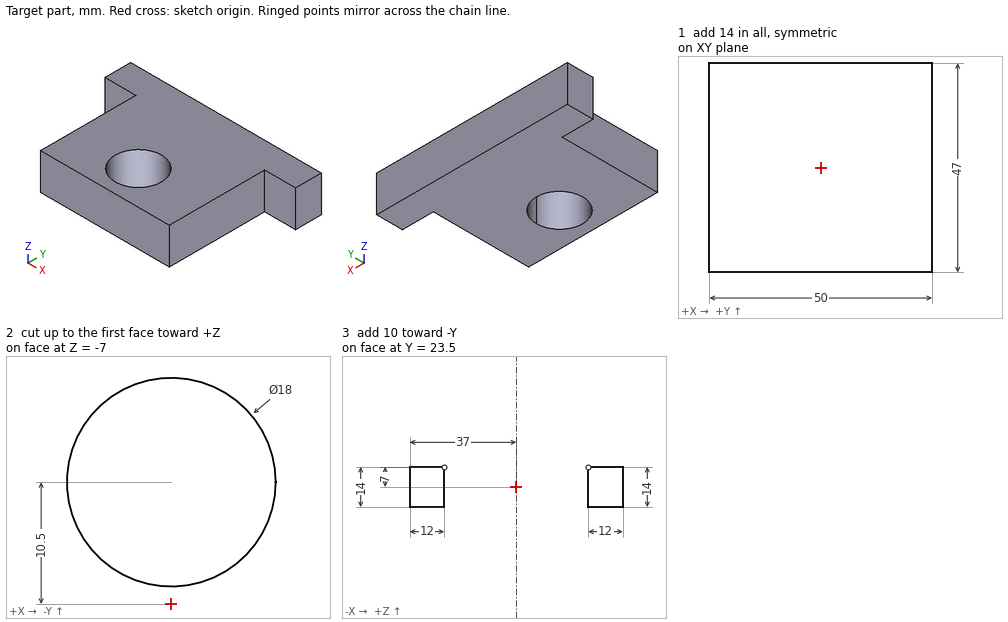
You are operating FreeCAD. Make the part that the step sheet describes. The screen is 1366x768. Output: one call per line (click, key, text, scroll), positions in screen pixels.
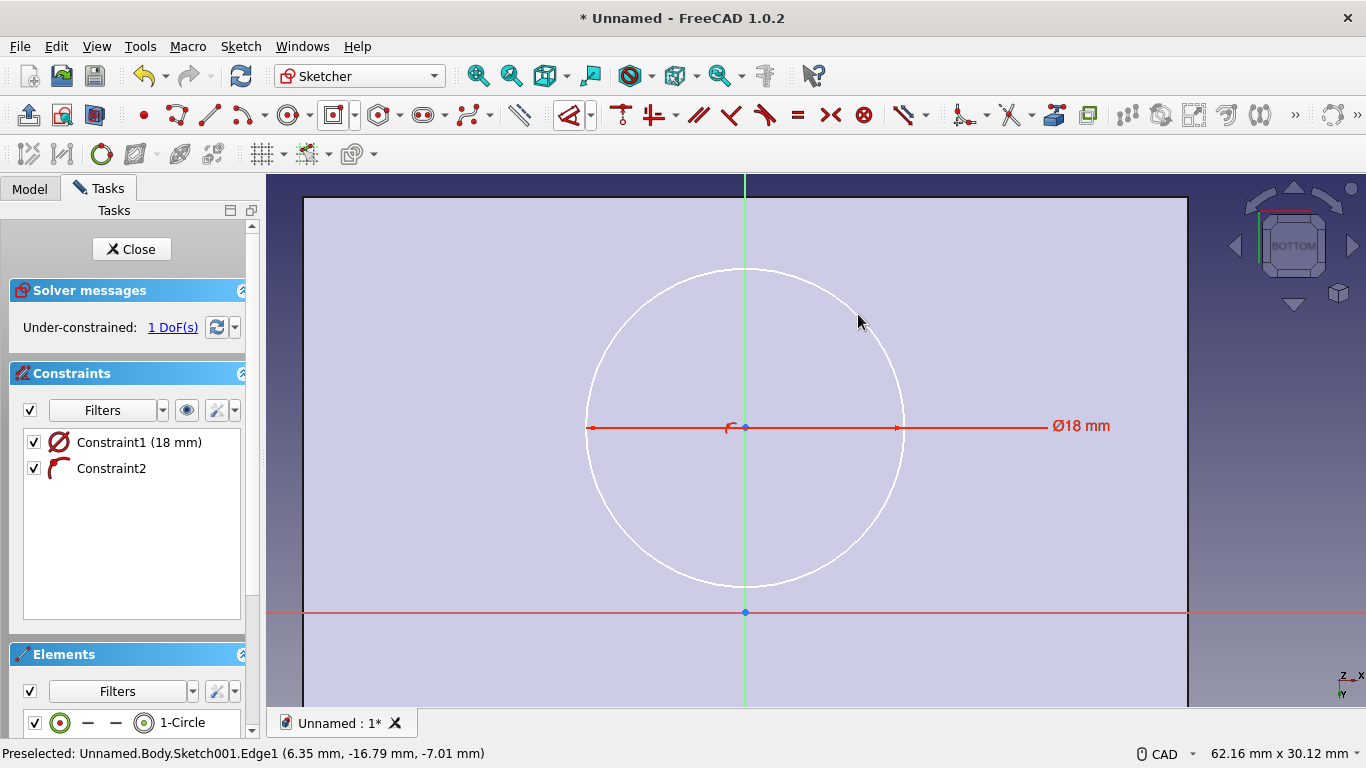
click(745, 428)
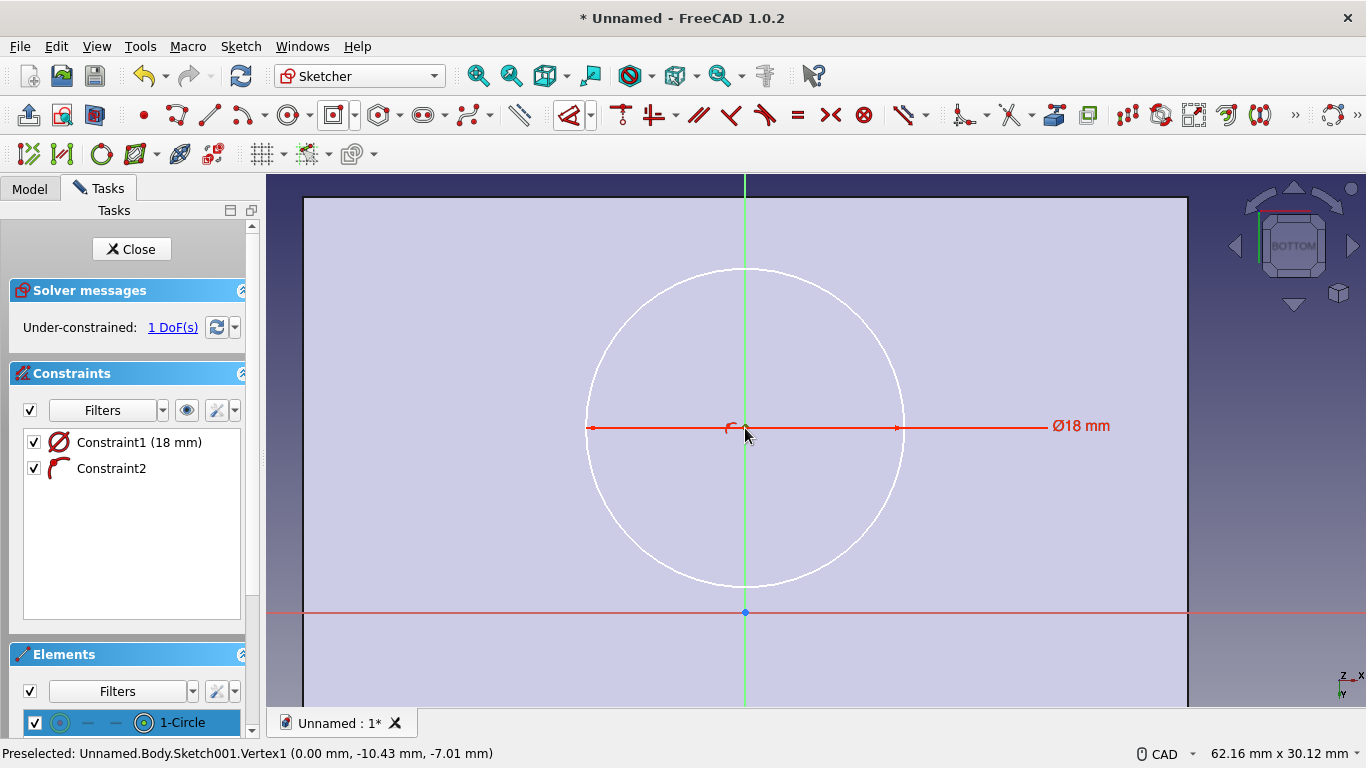
click(590, 116)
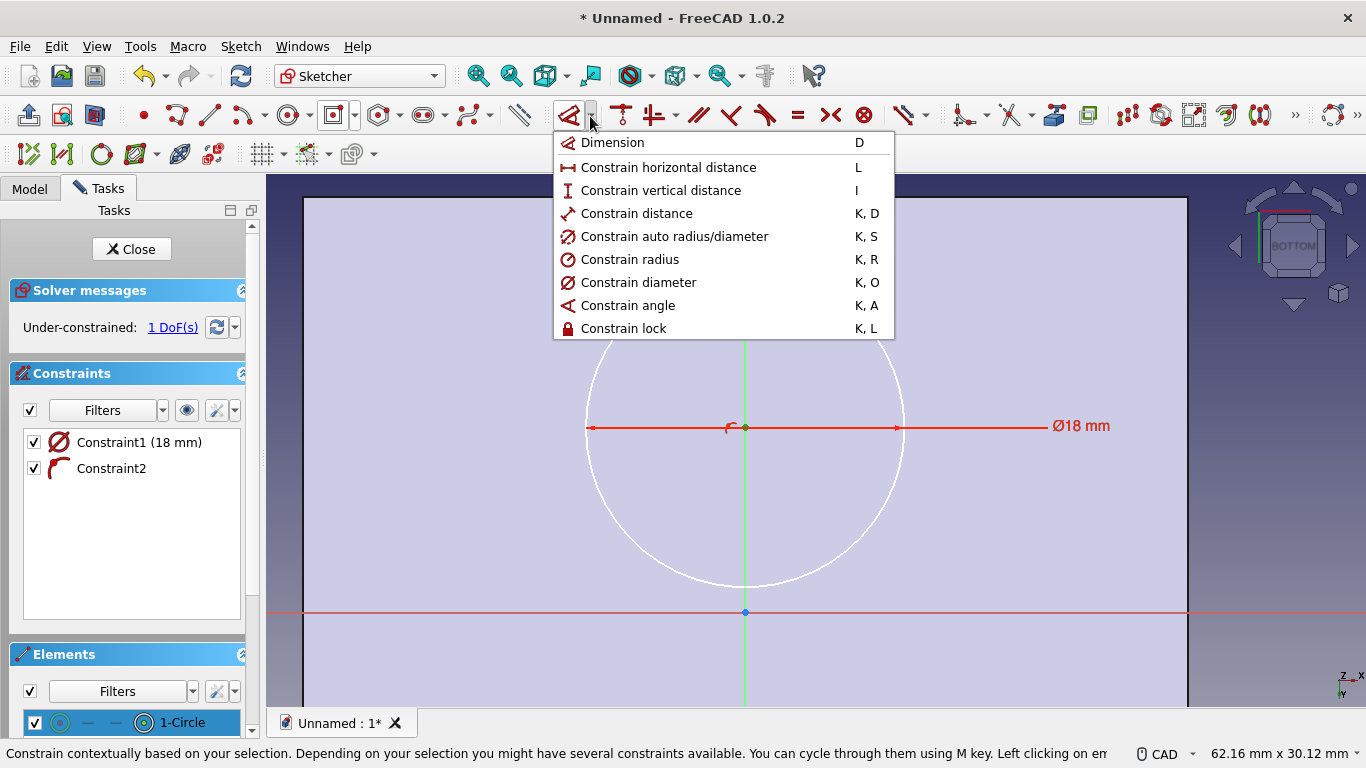
click(724, 190)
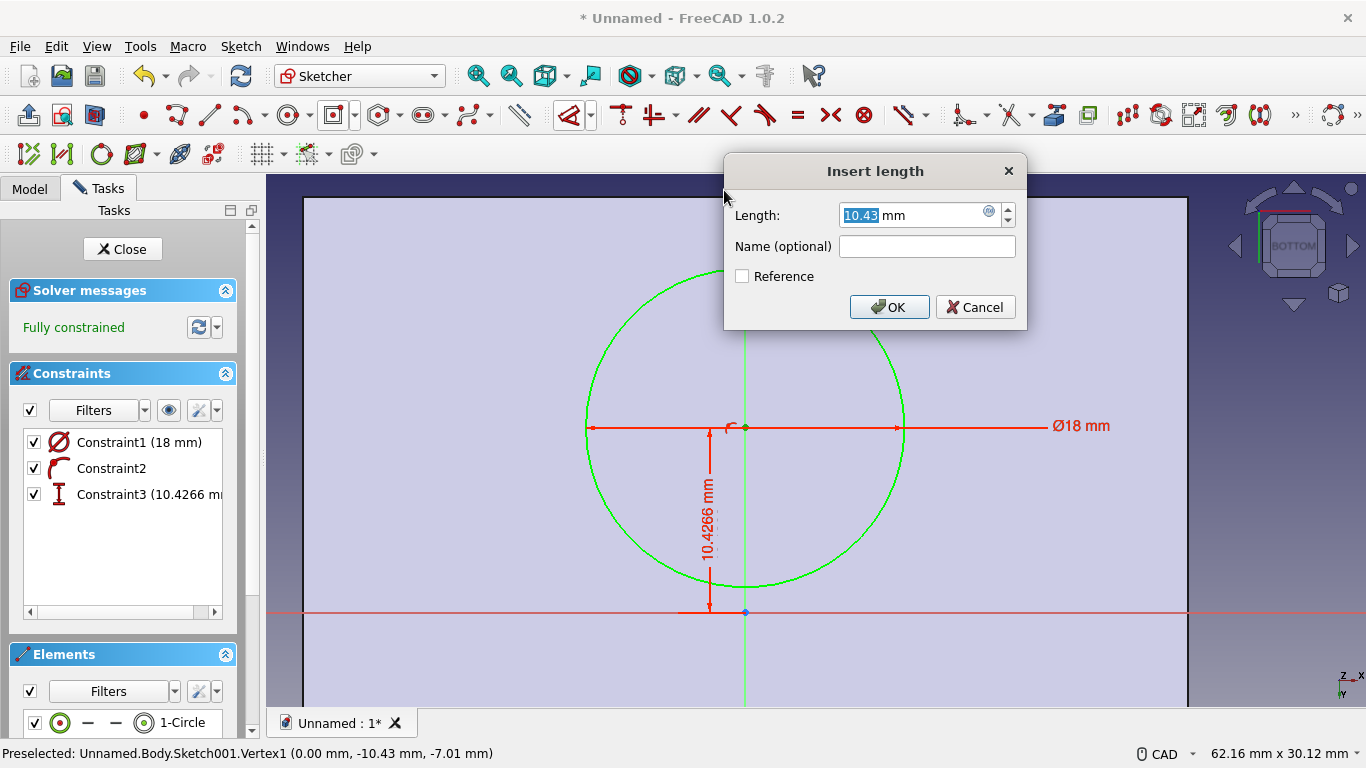
text(10.5)
key(Return)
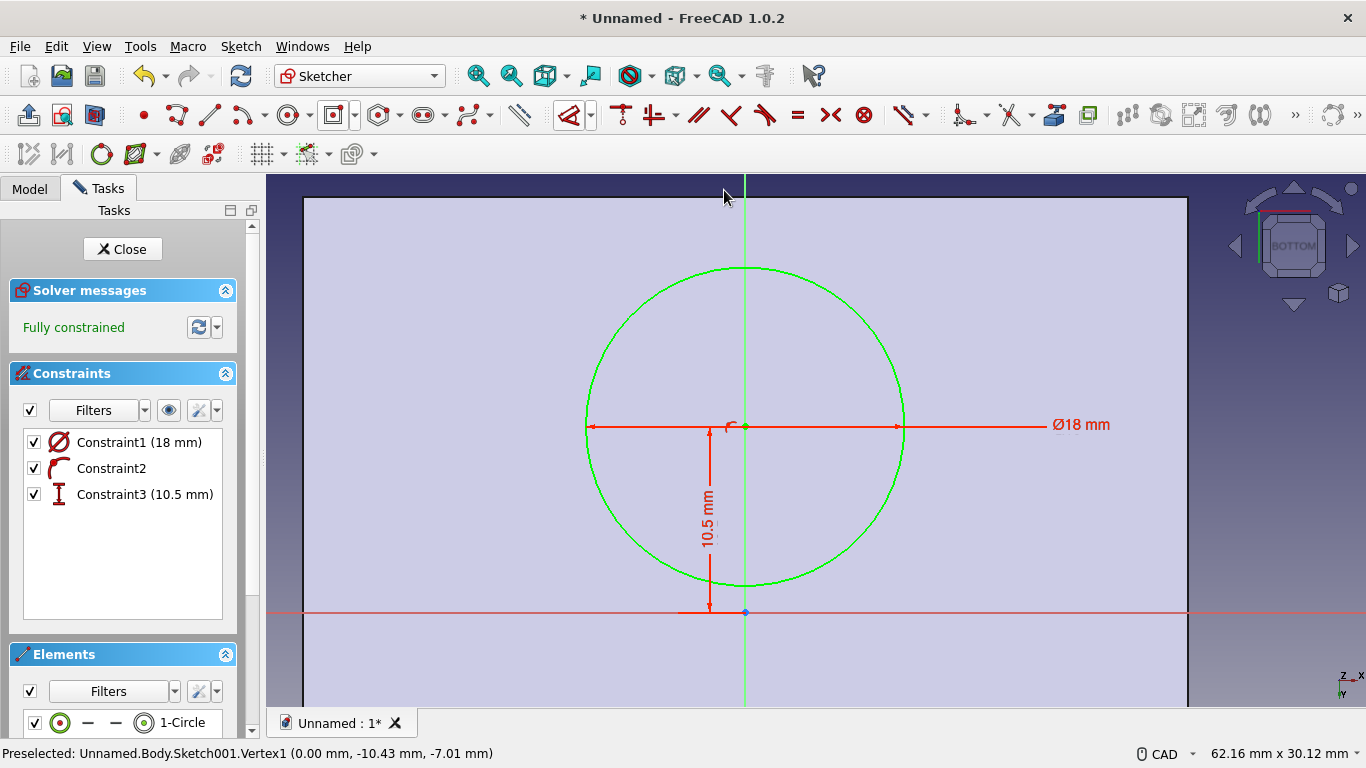
click(123, 249)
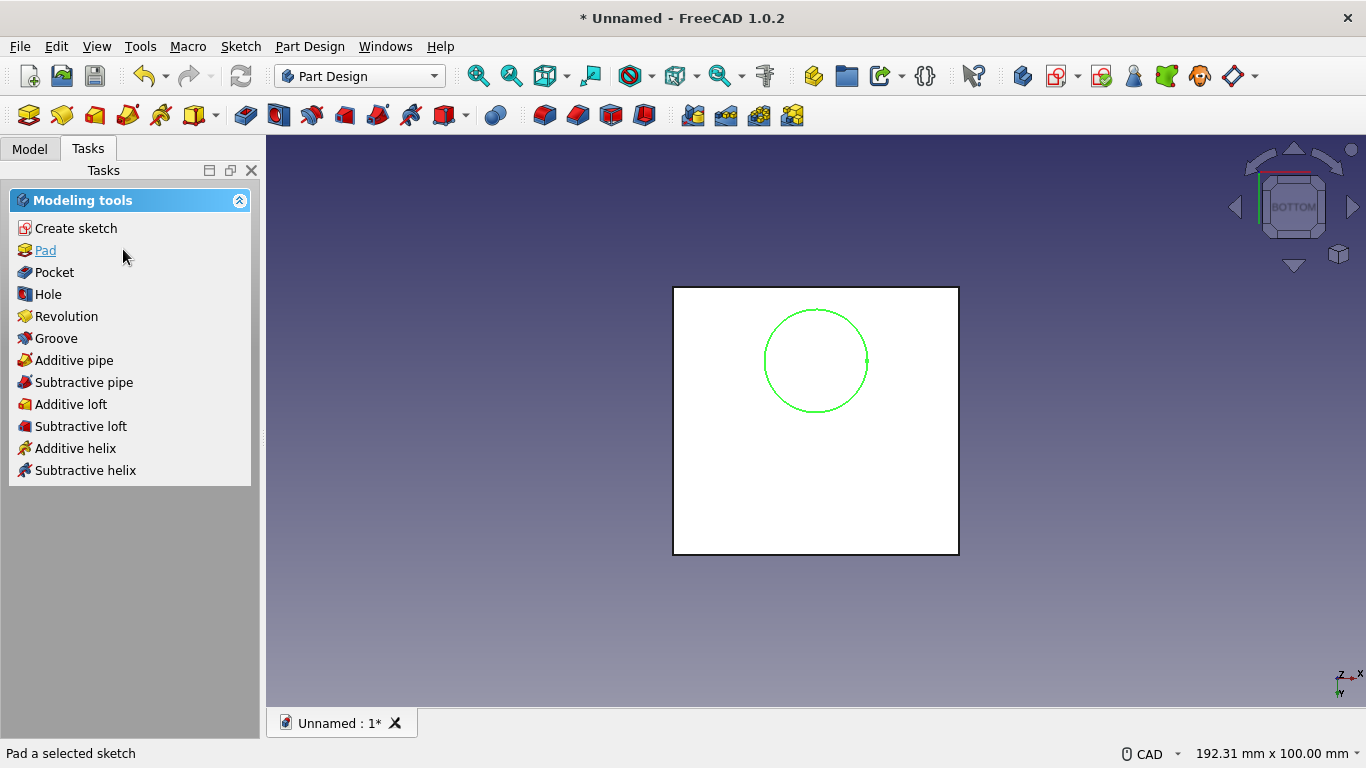
click(246, 116)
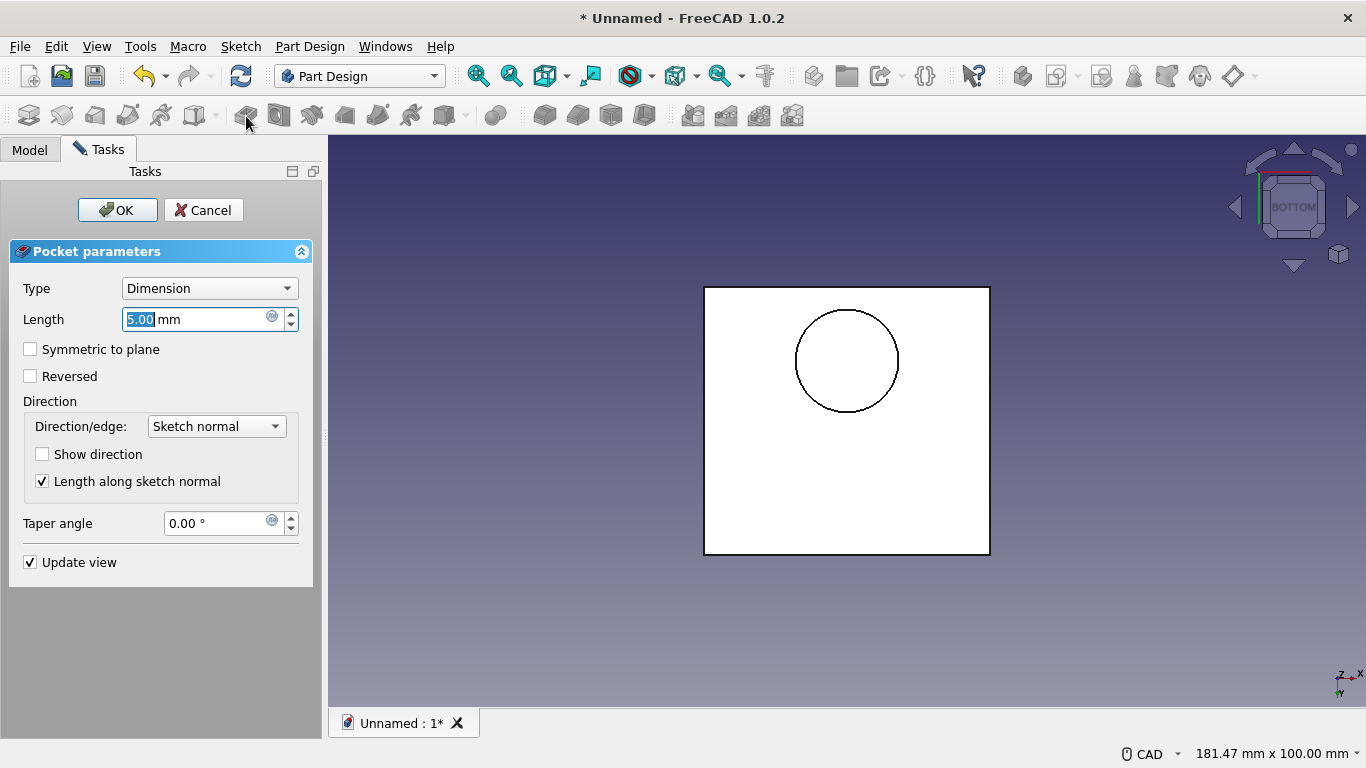
click(210, 288)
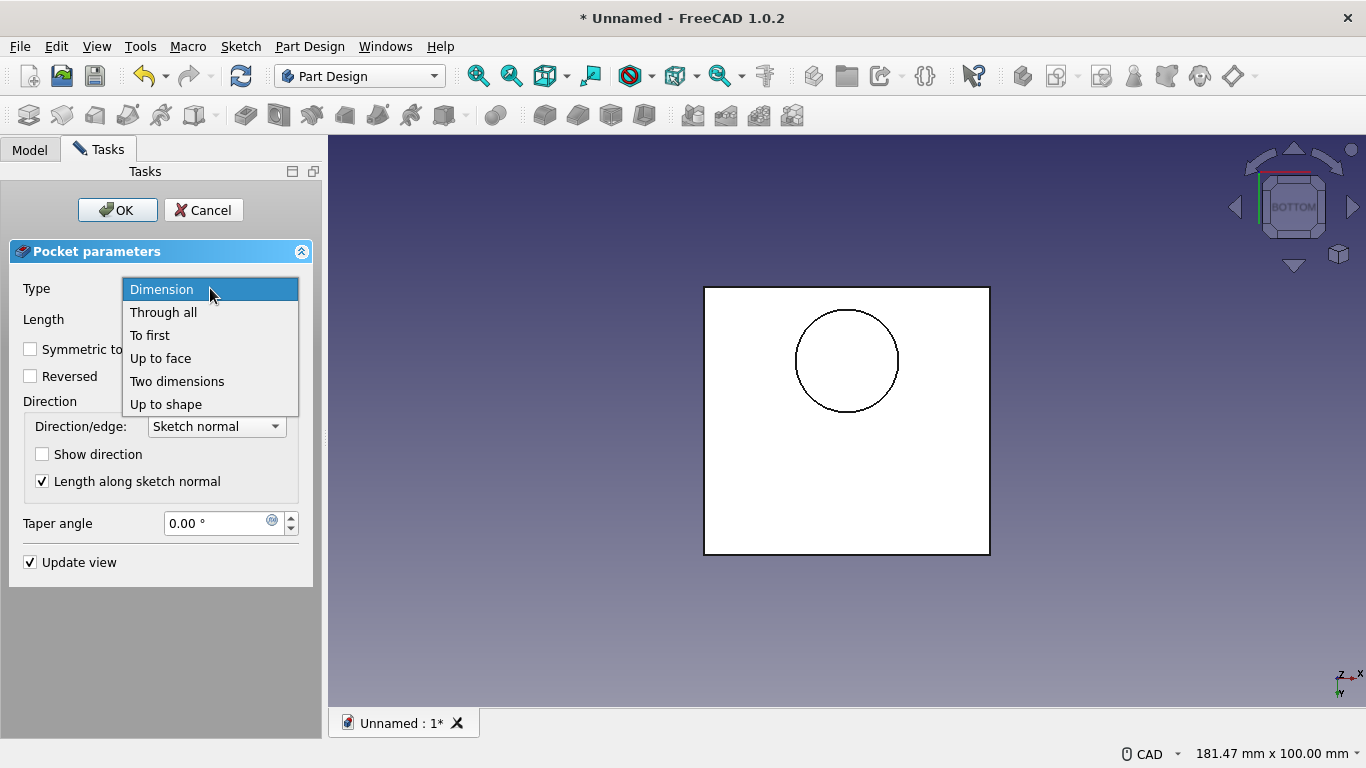
click(208, 336)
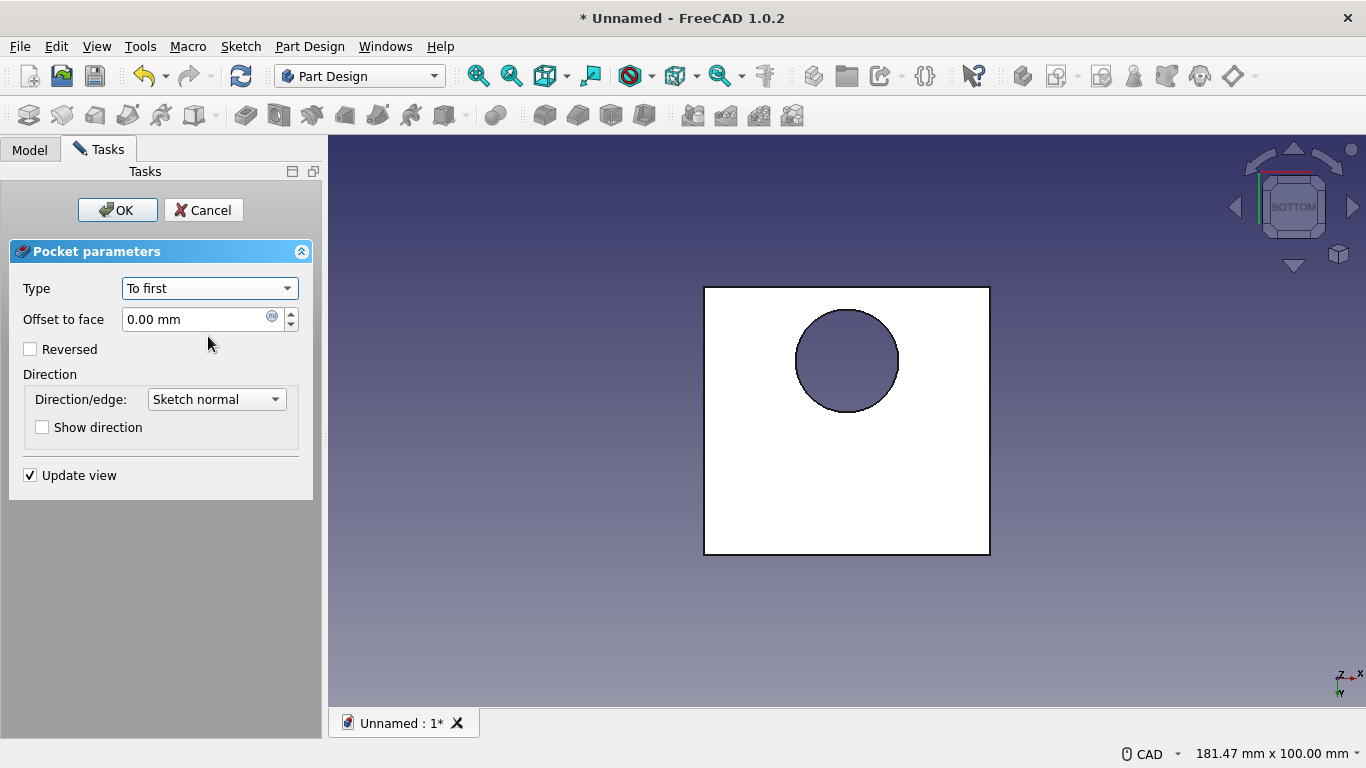
click(118, 210)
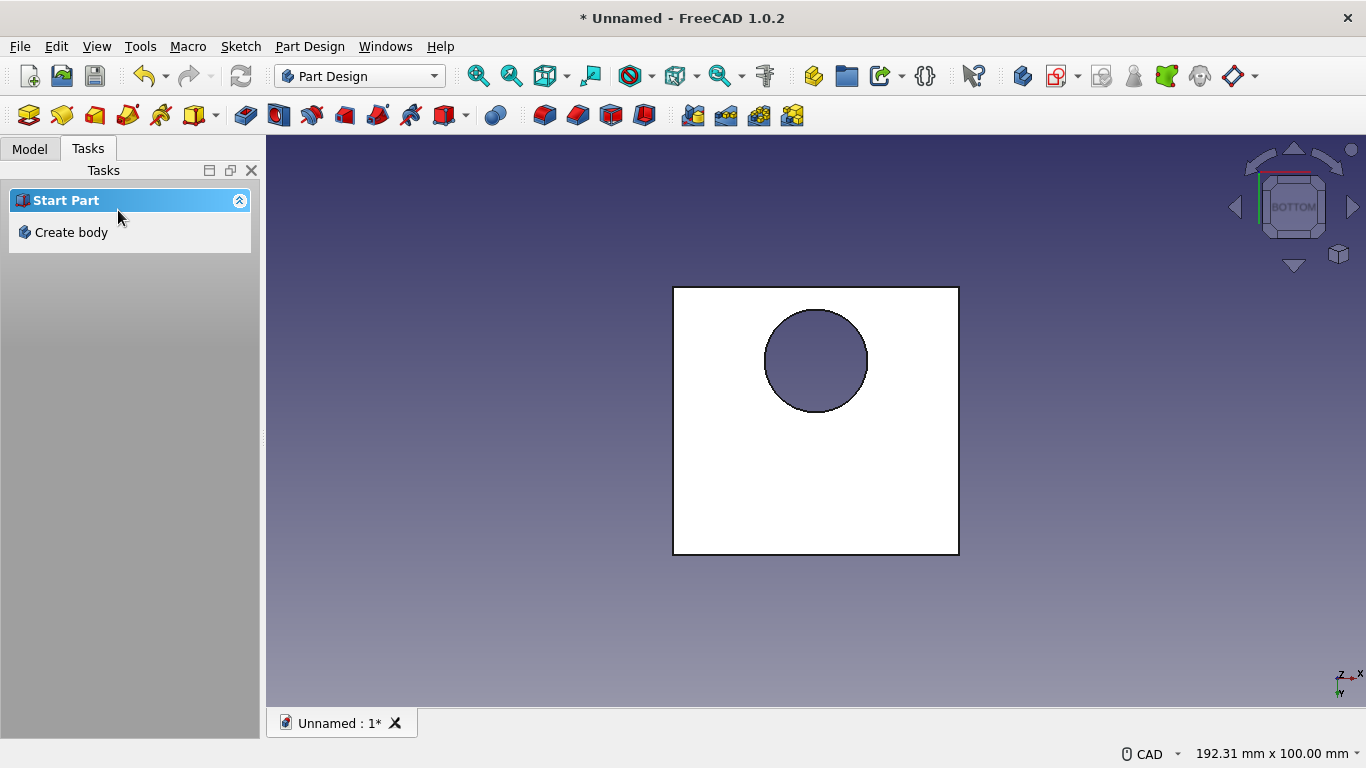
key(4)